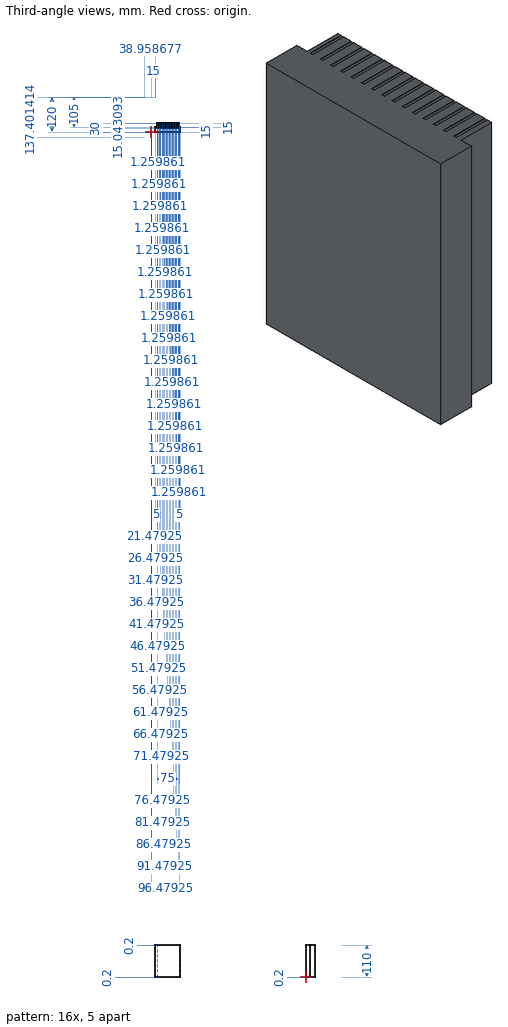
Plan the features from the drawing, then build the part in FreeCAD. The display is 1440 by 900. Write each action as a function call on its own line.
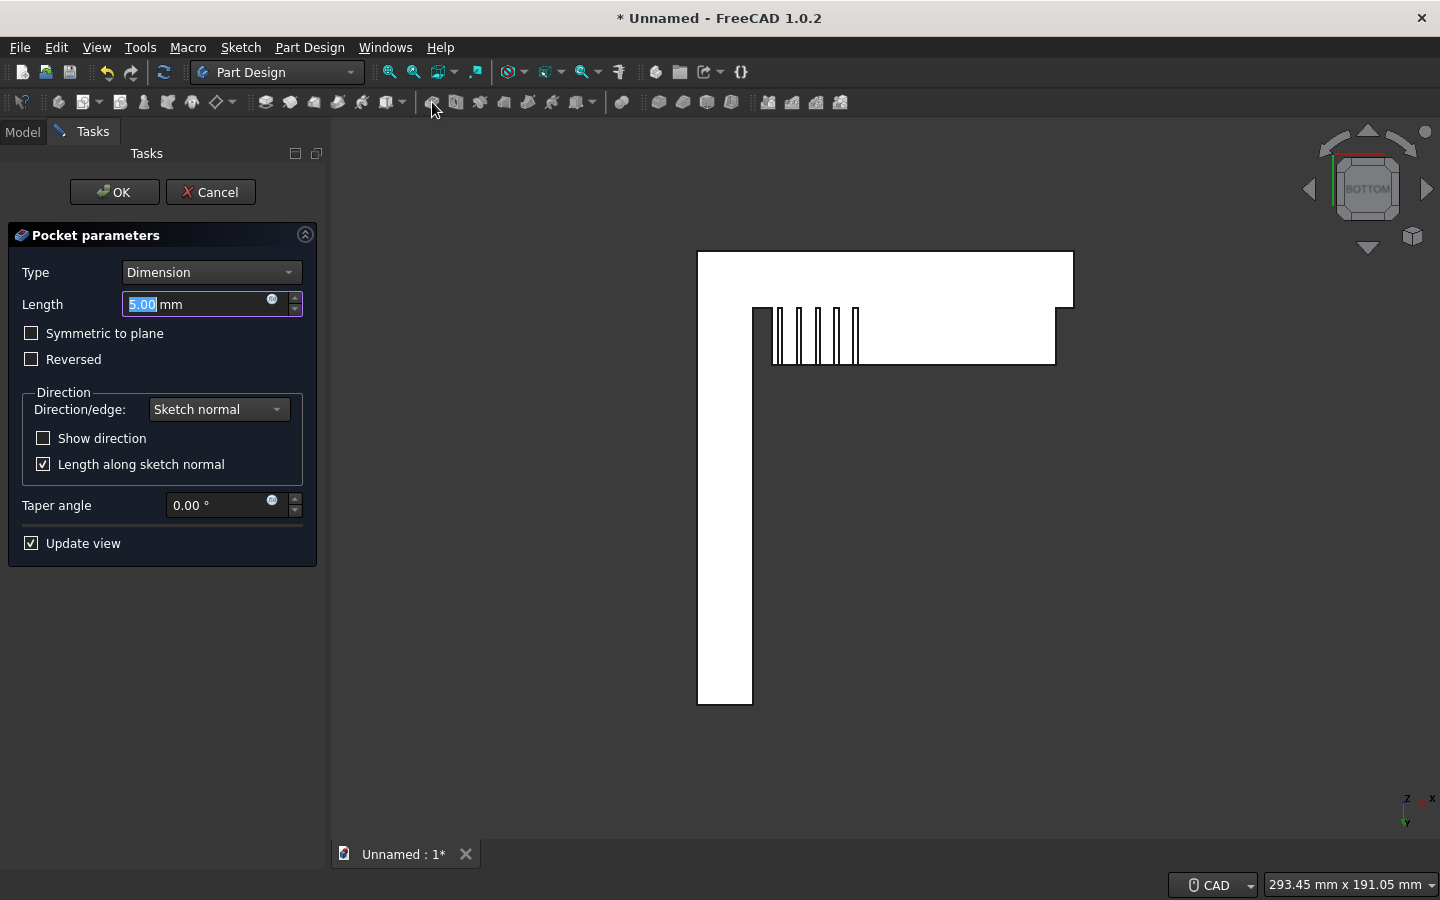
text(0.2)
key(Tab)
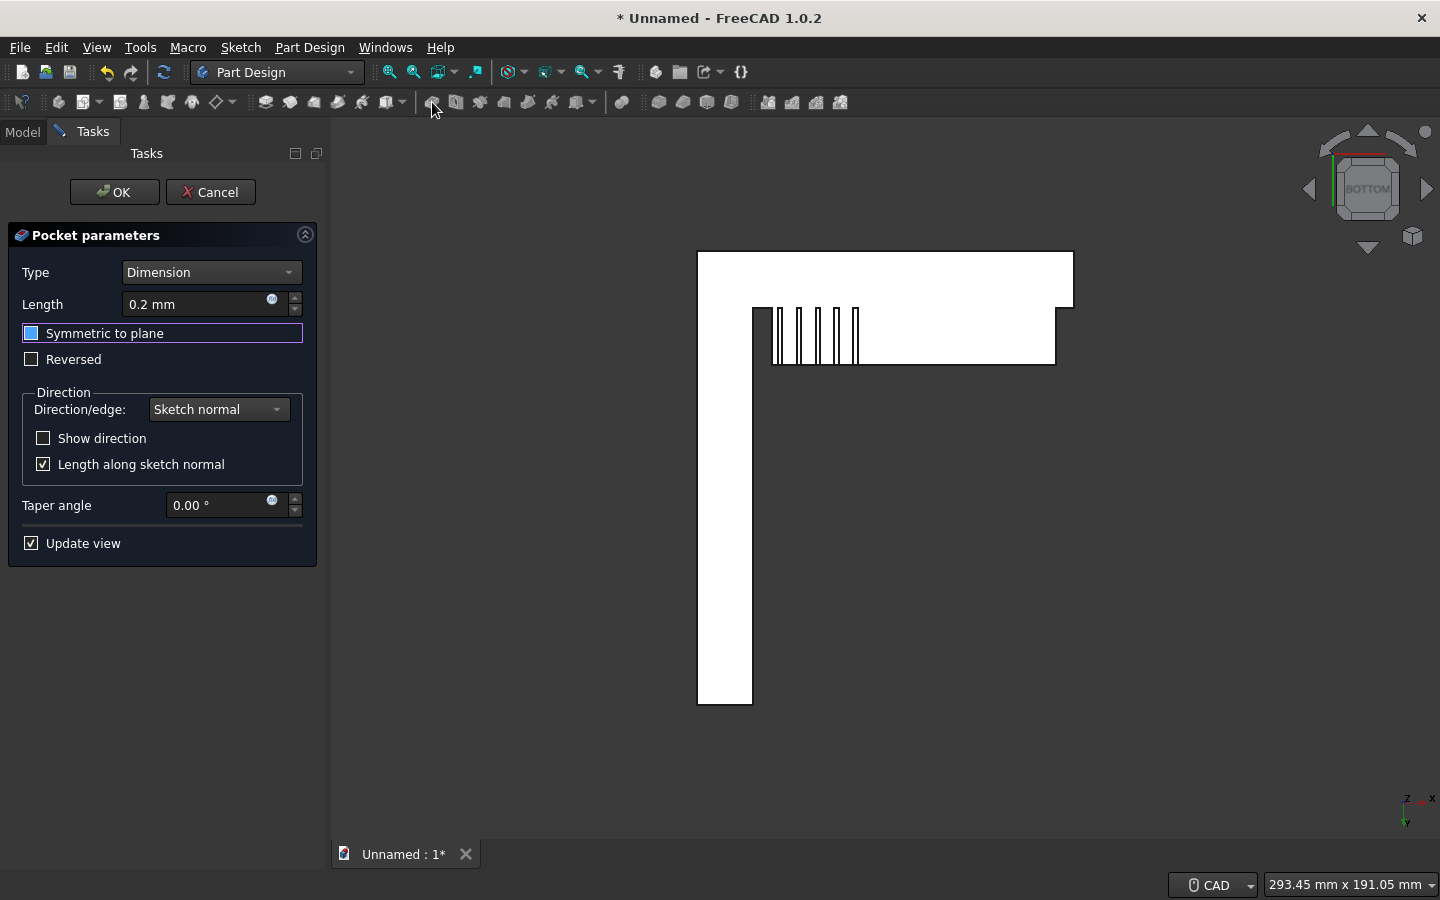
click(30, 359)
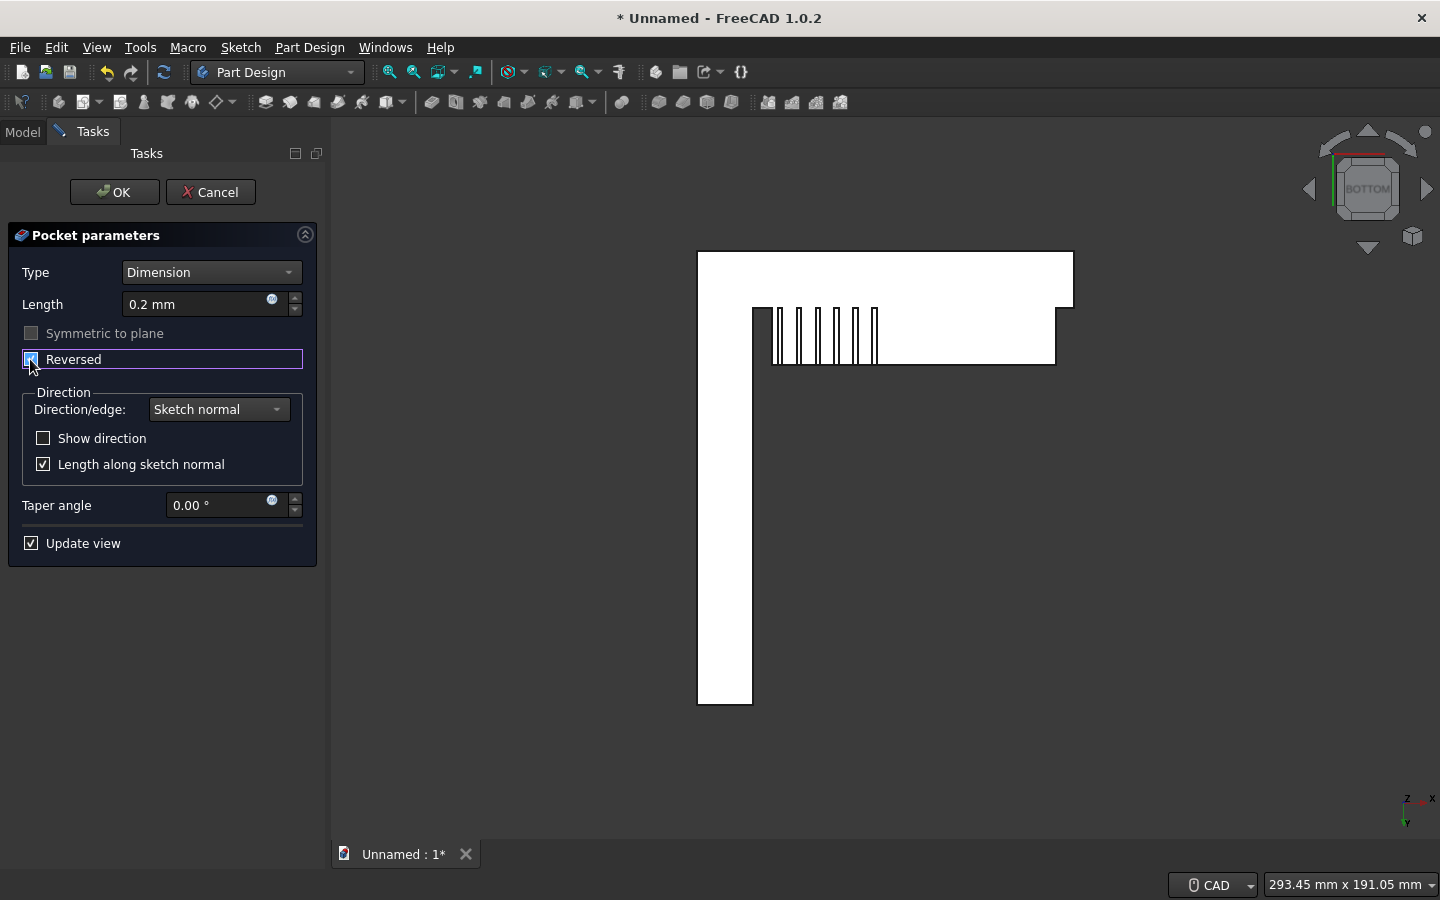
click(115, 192)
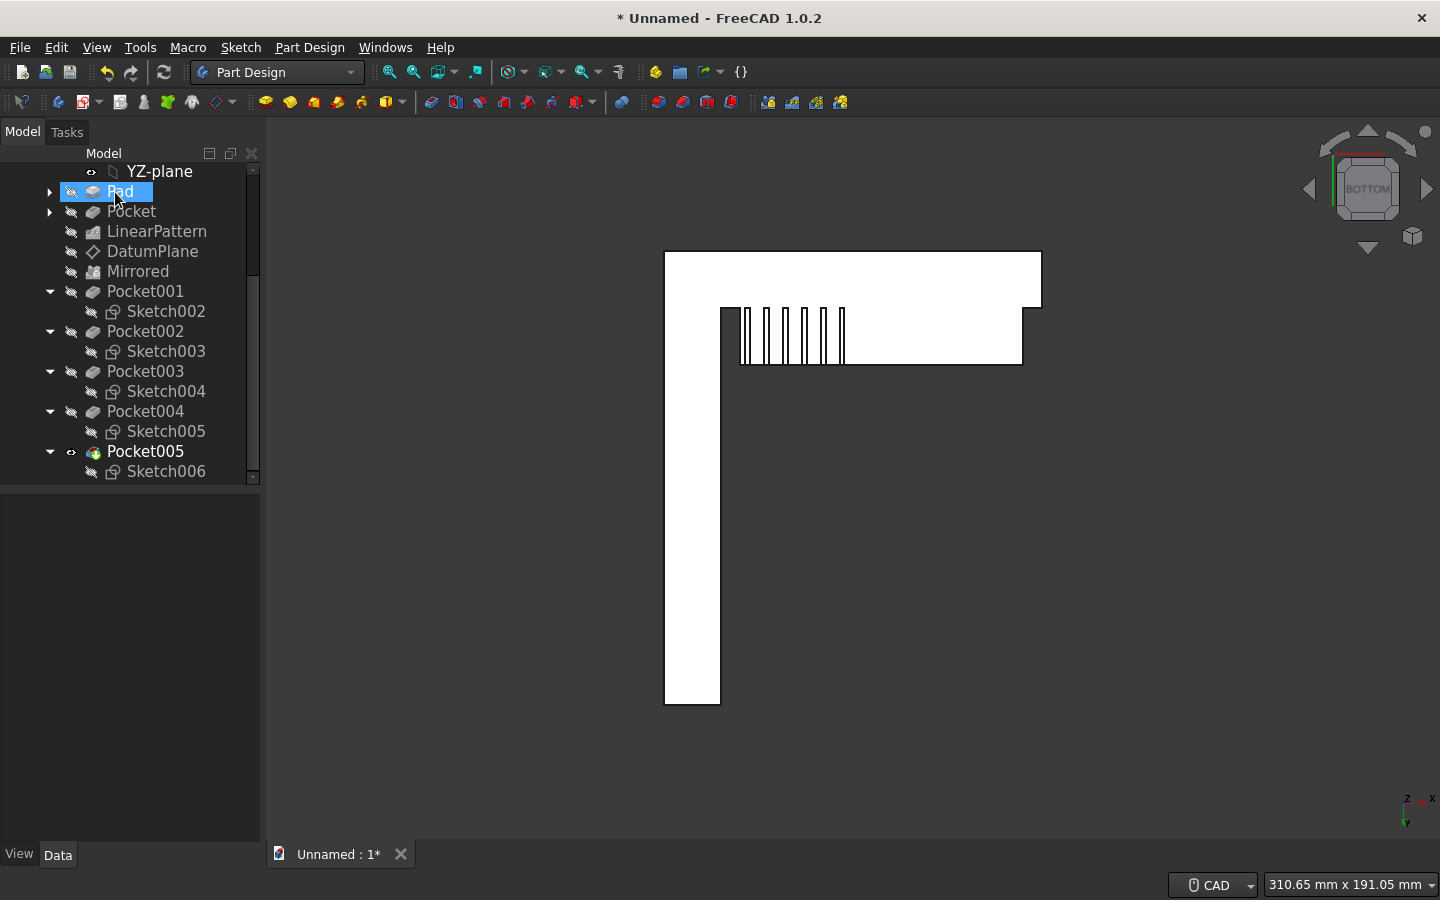
click(84, 102)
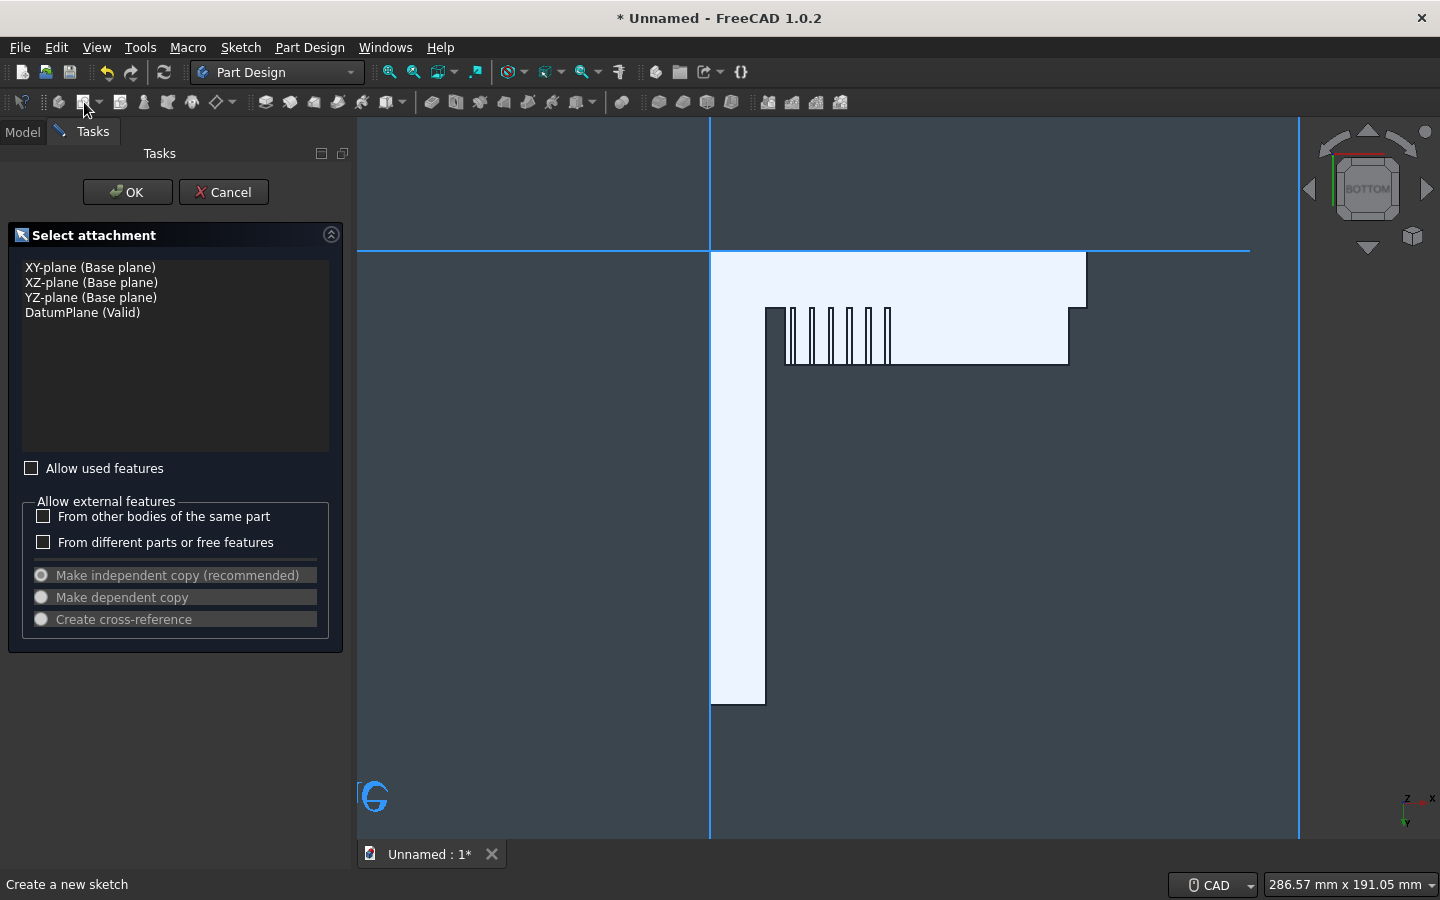
click(82, 268)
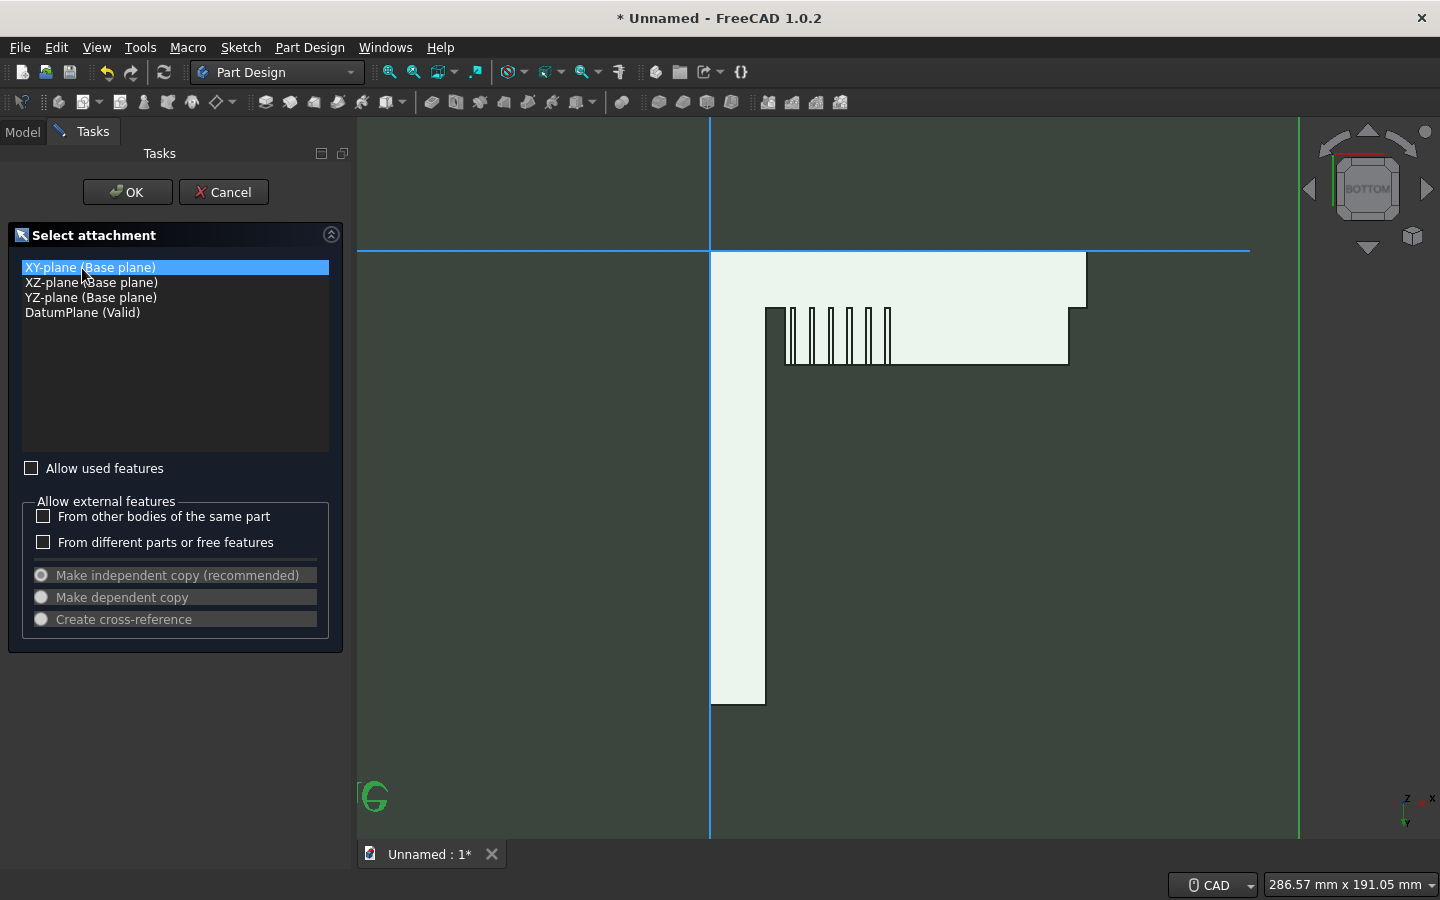
click(128, 192)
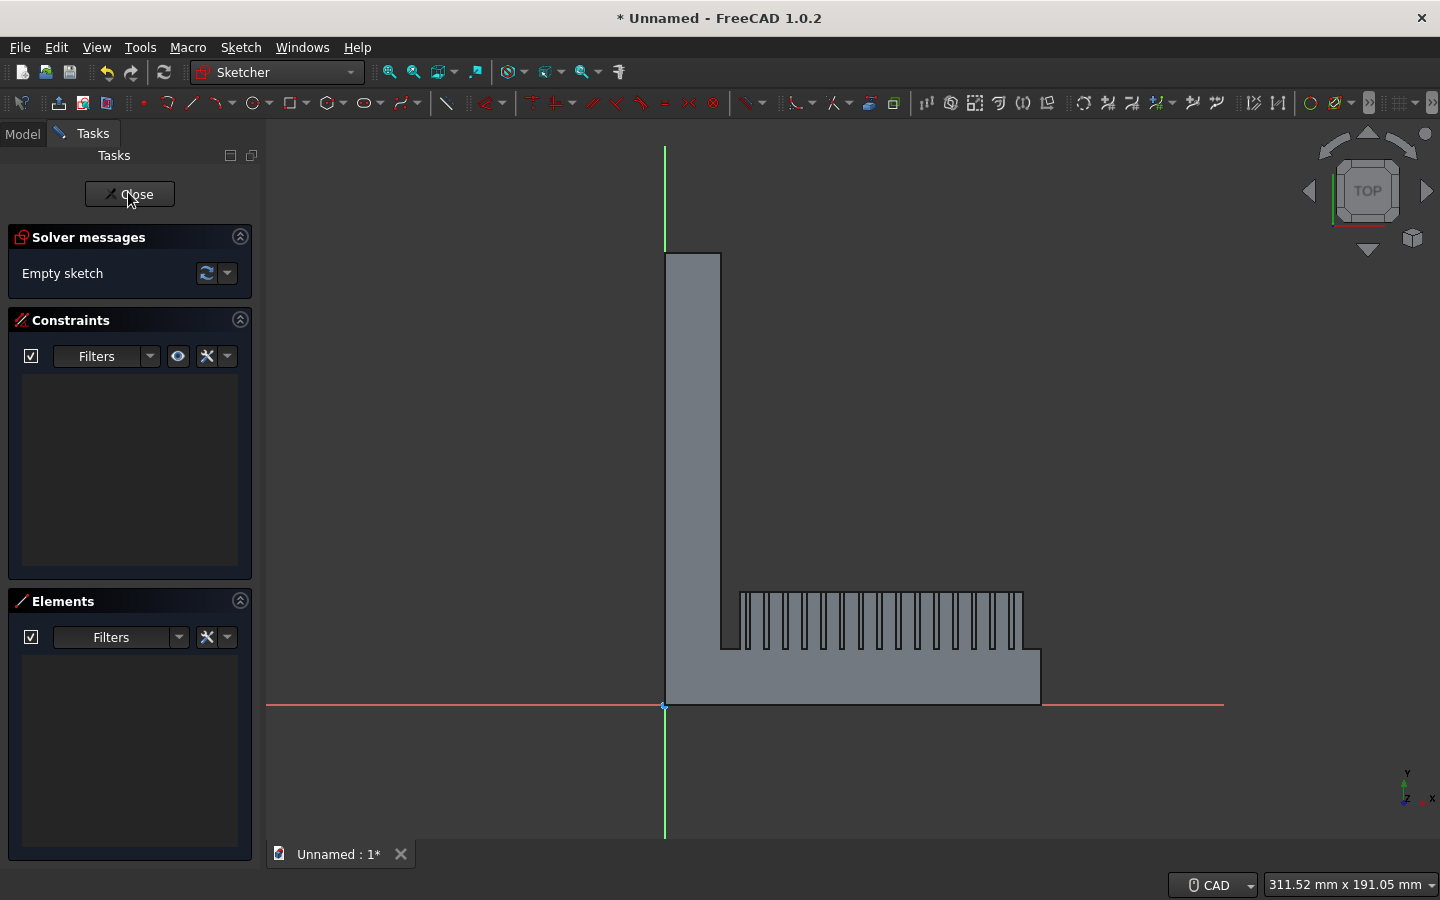
key(q)
key(s)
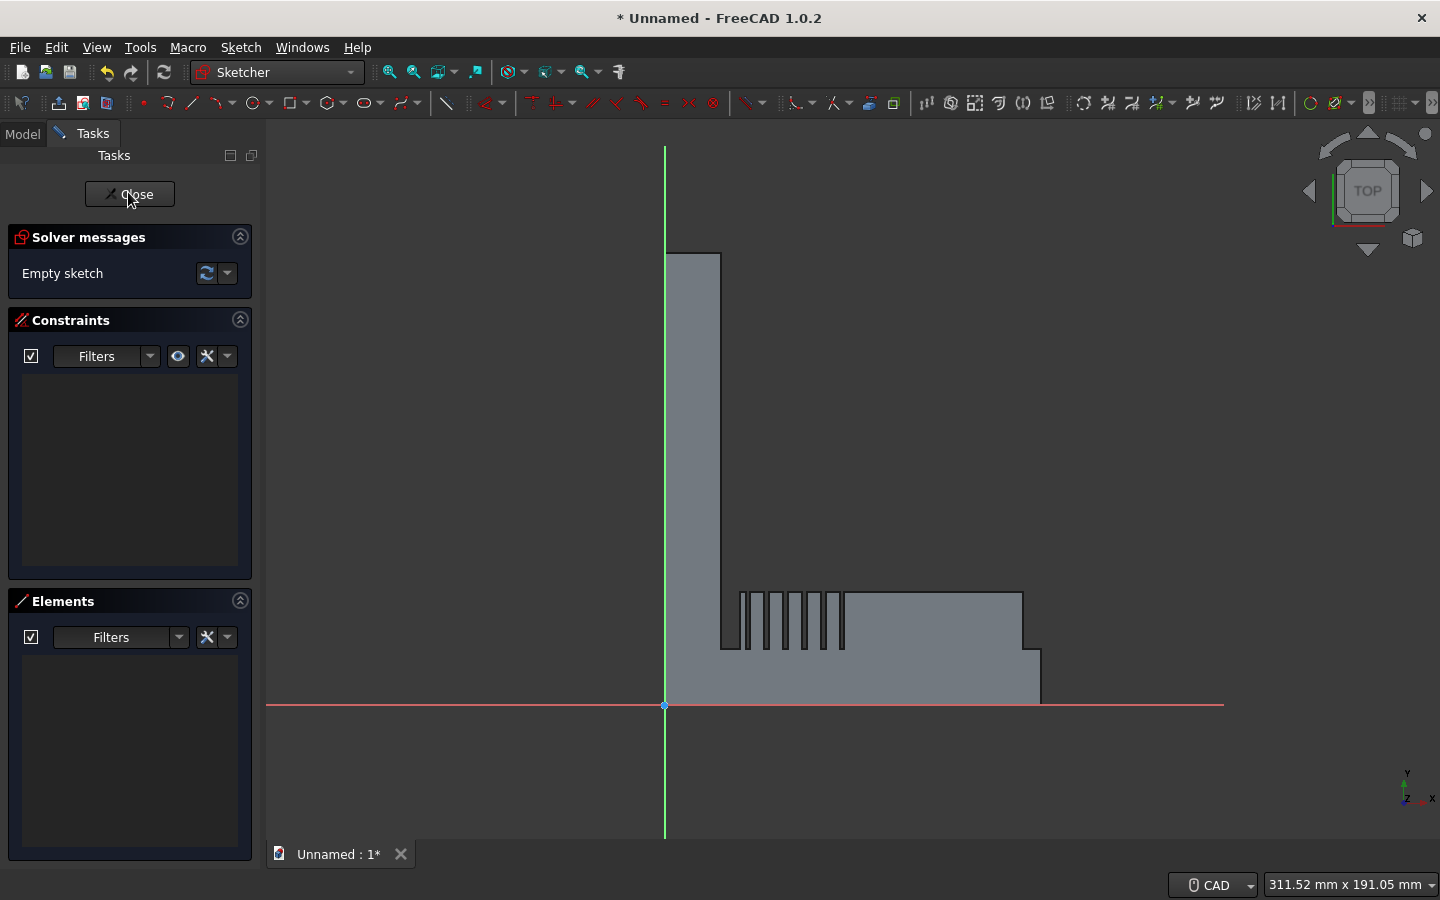
scroll(870, 638, up, 11)